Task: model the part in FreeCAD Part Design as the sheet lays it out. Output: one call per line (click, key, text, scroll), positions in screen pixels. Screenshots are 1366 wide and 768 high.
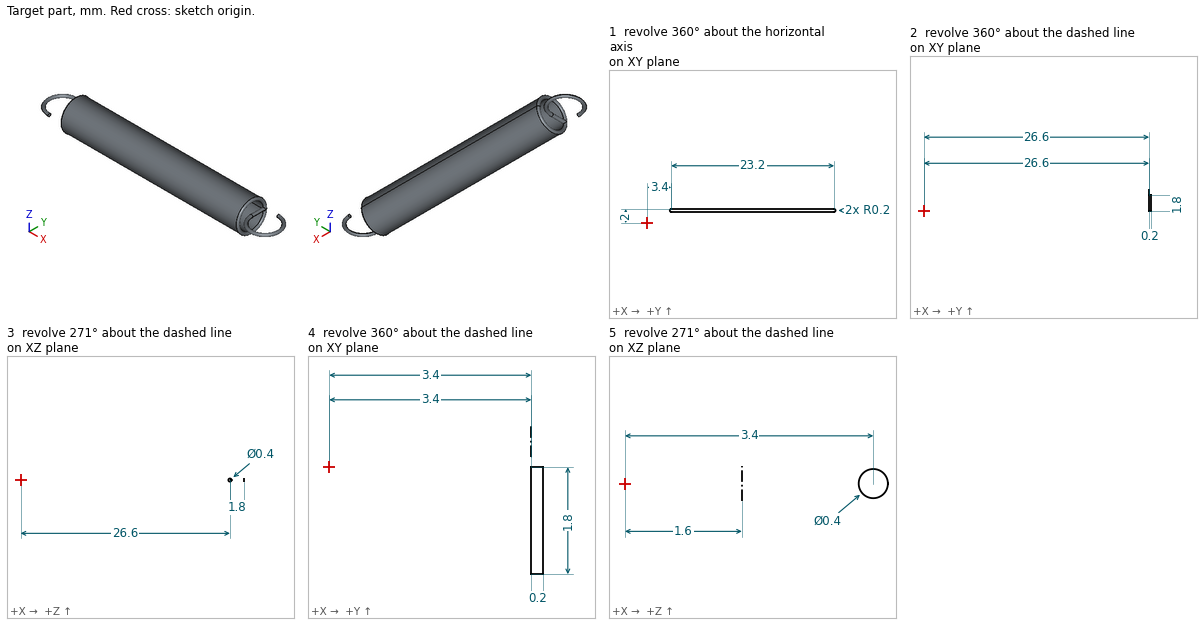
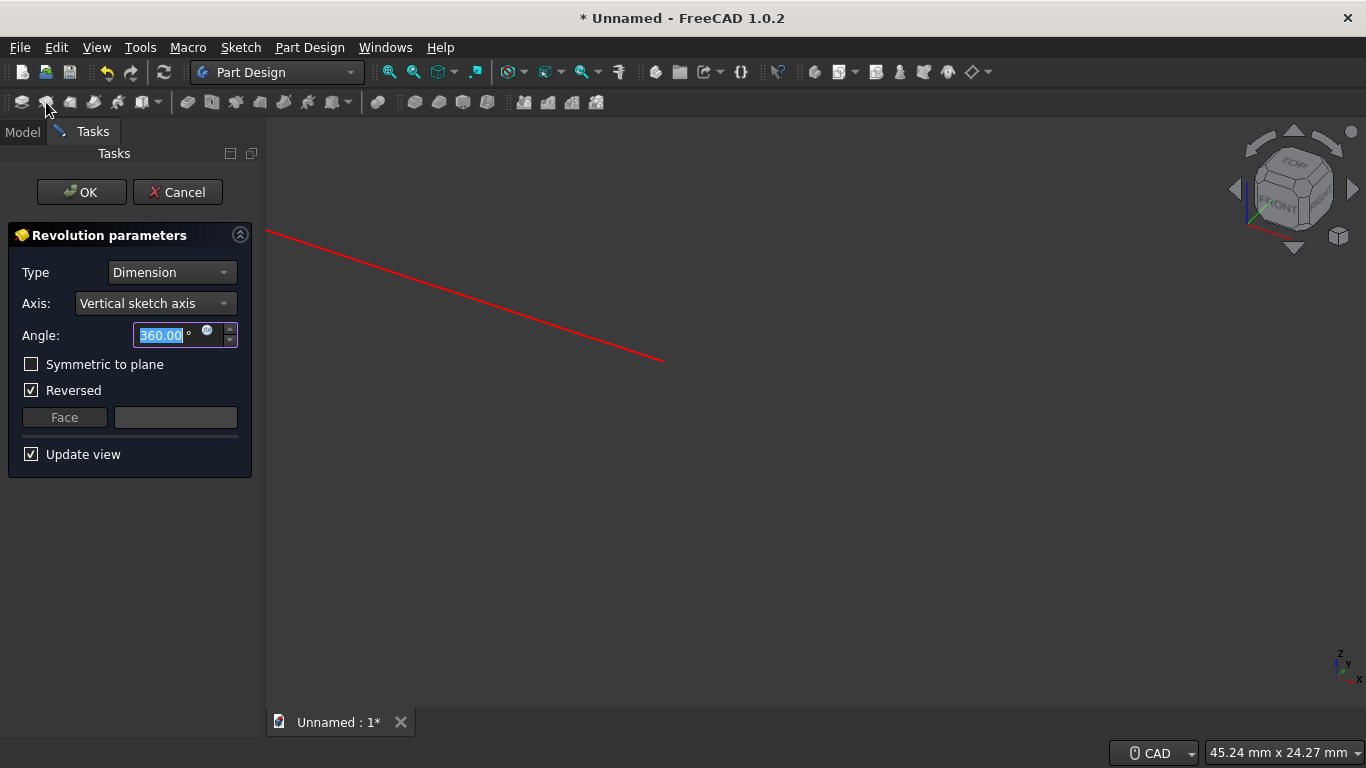
click(156, 304)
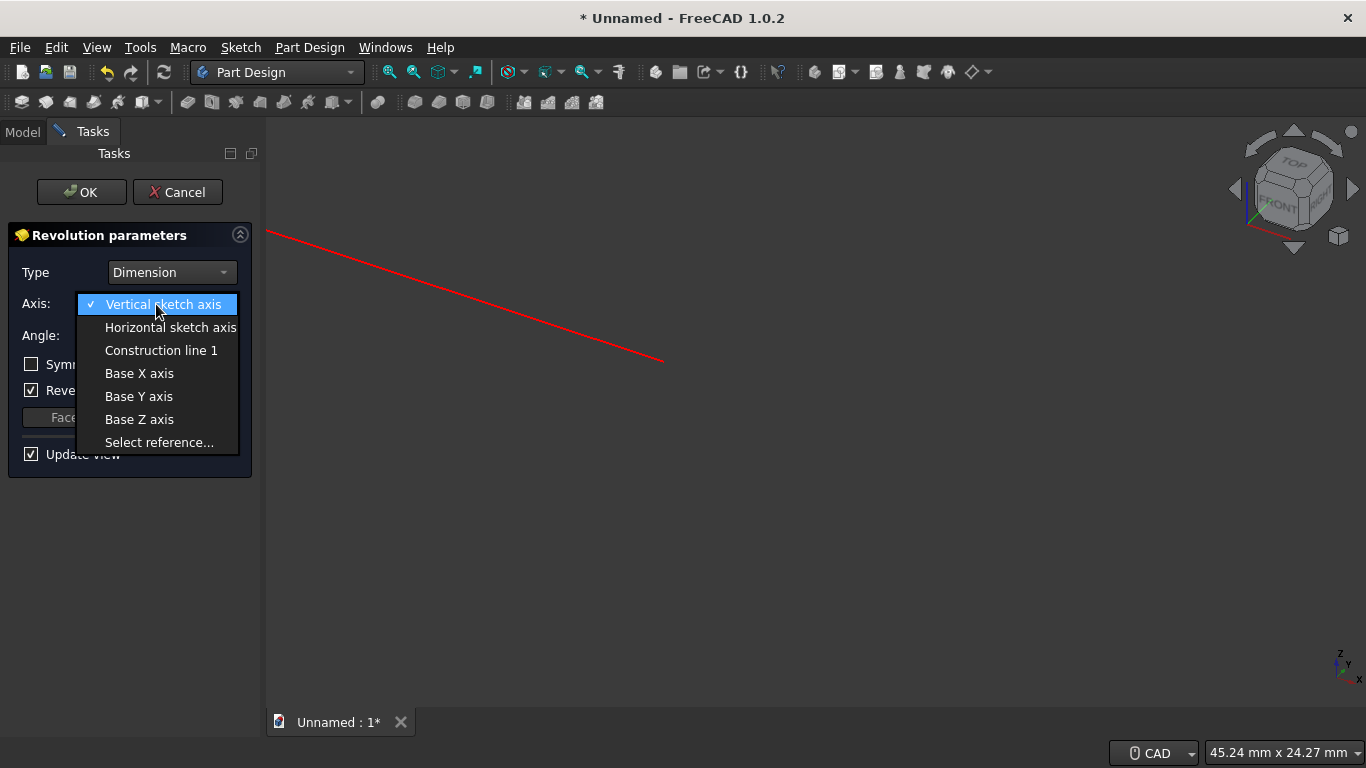
click(156, 350)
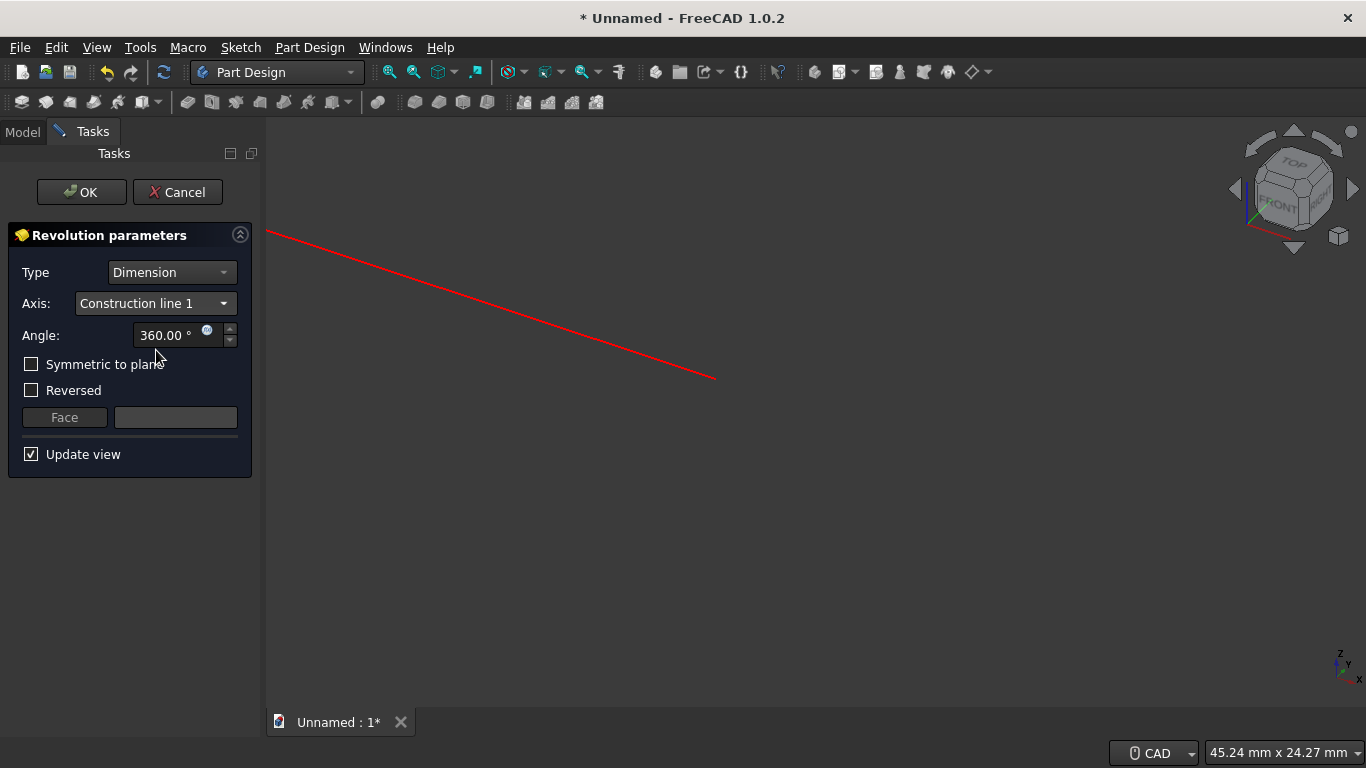
triple_click(178, 335)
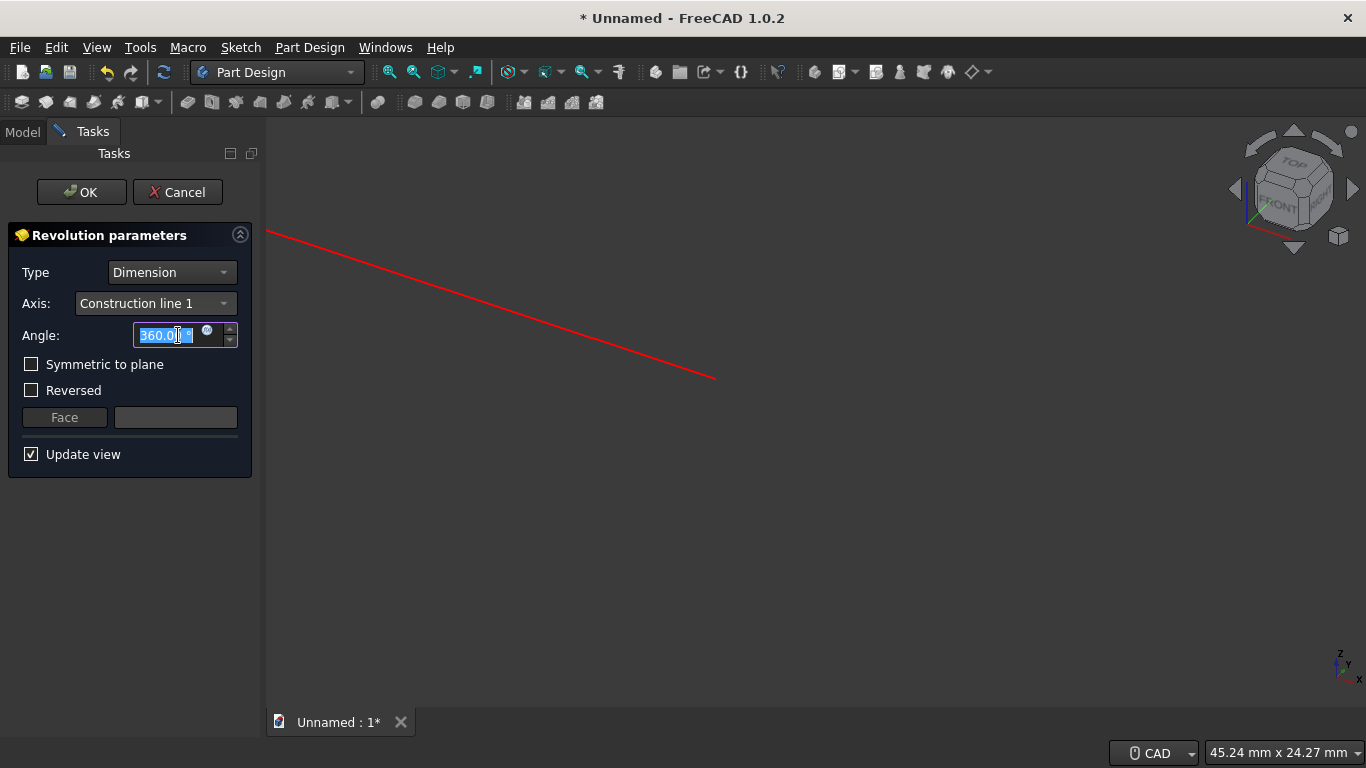
text(271)
key(Tab)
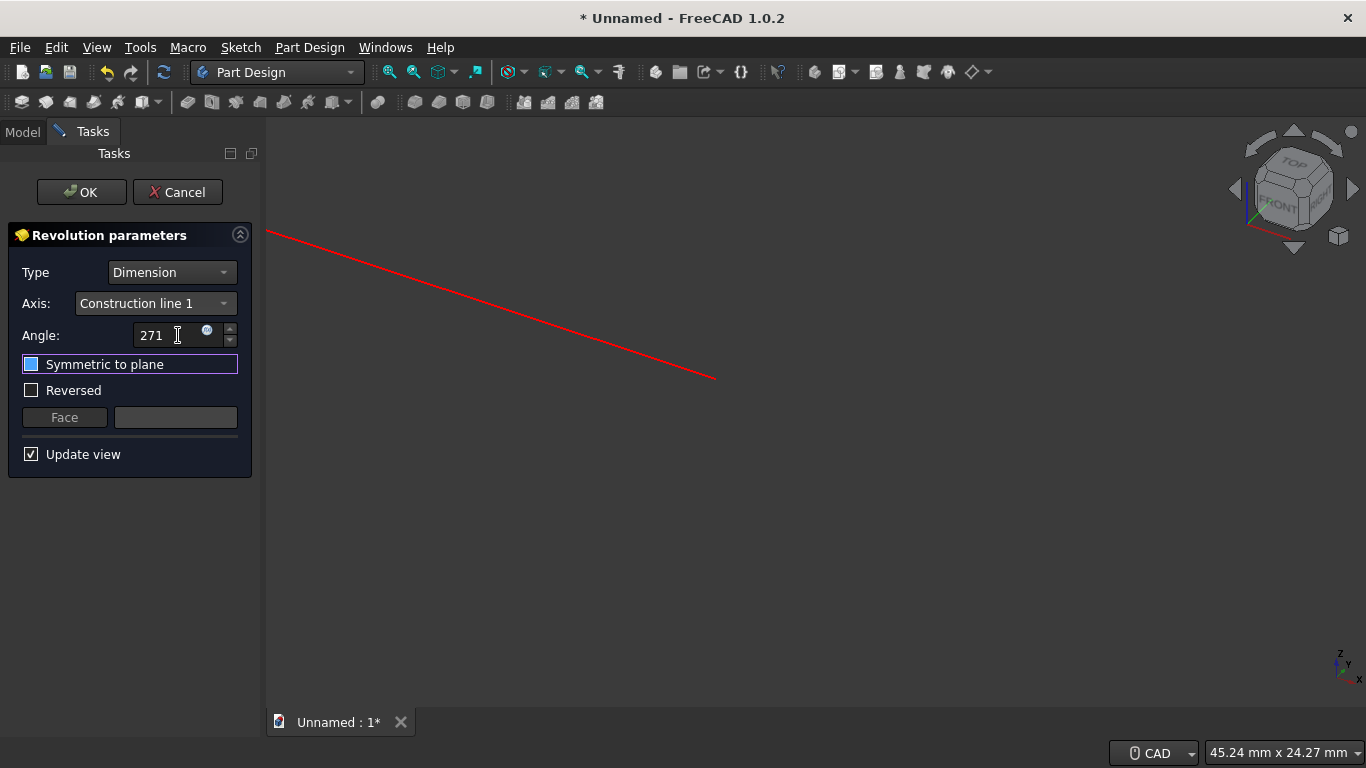
click(82, 192)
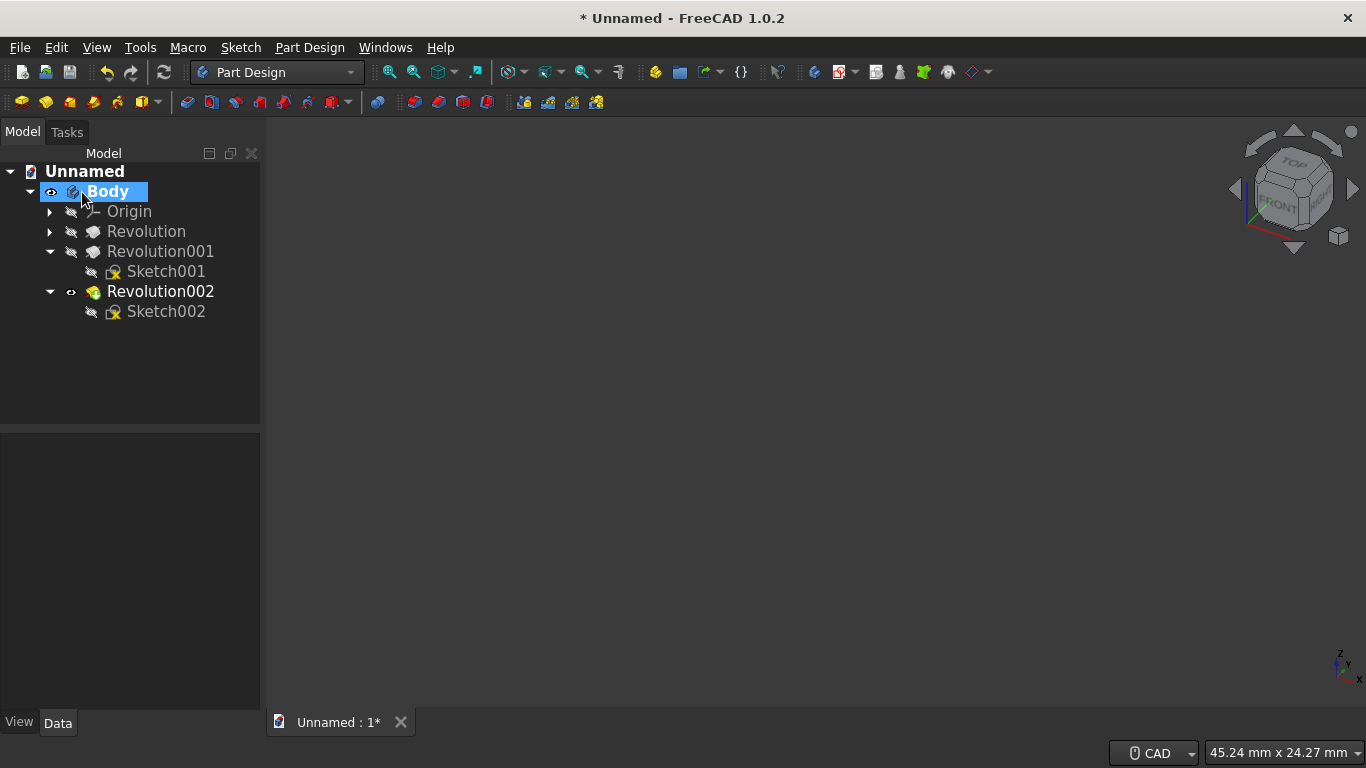
click(390, 72)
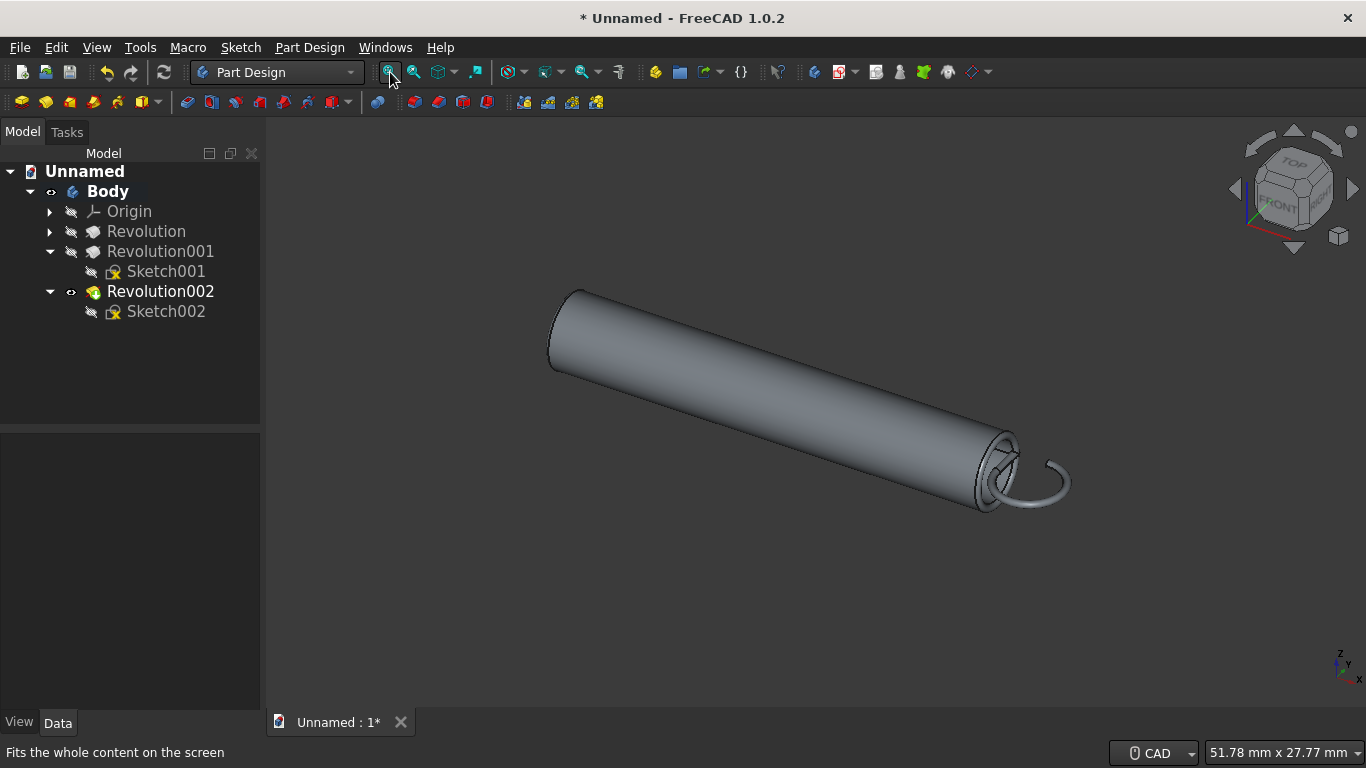
click(840, 72)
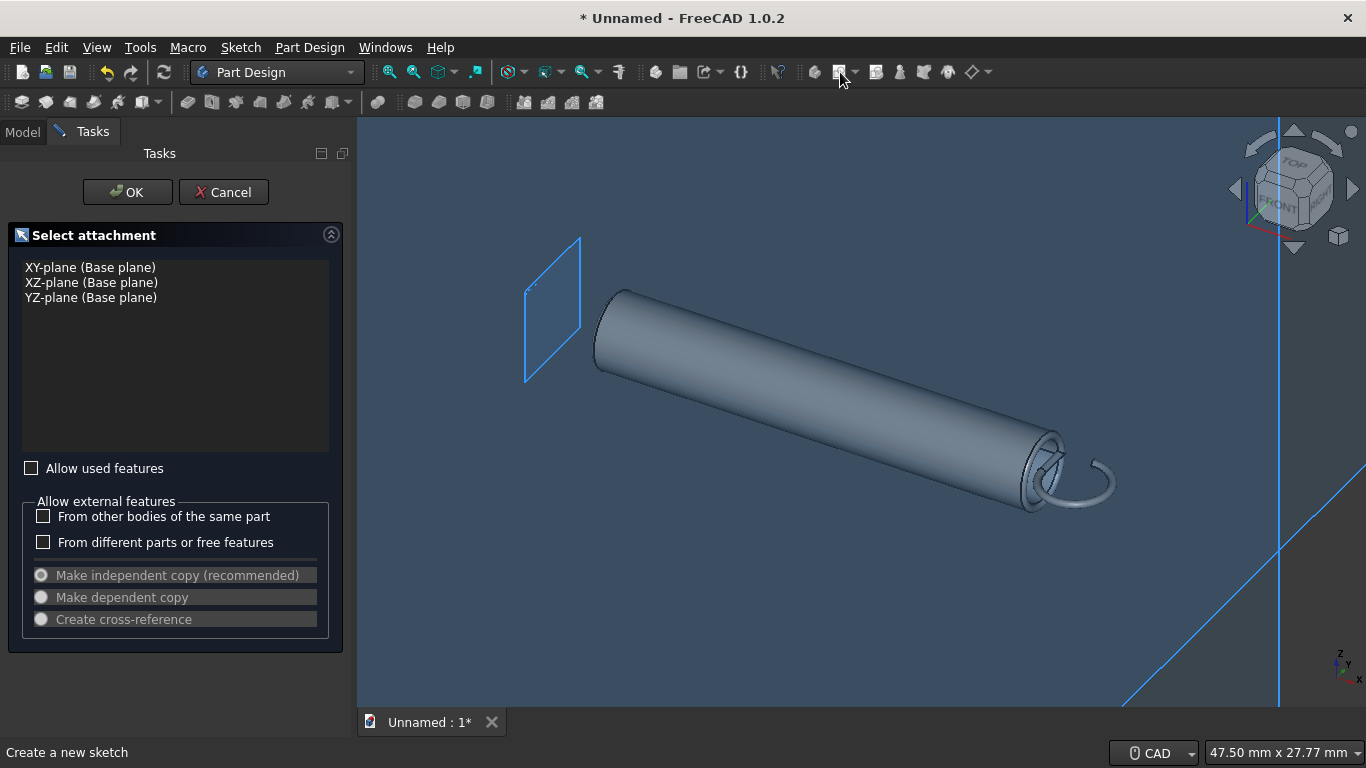
click(82, 268)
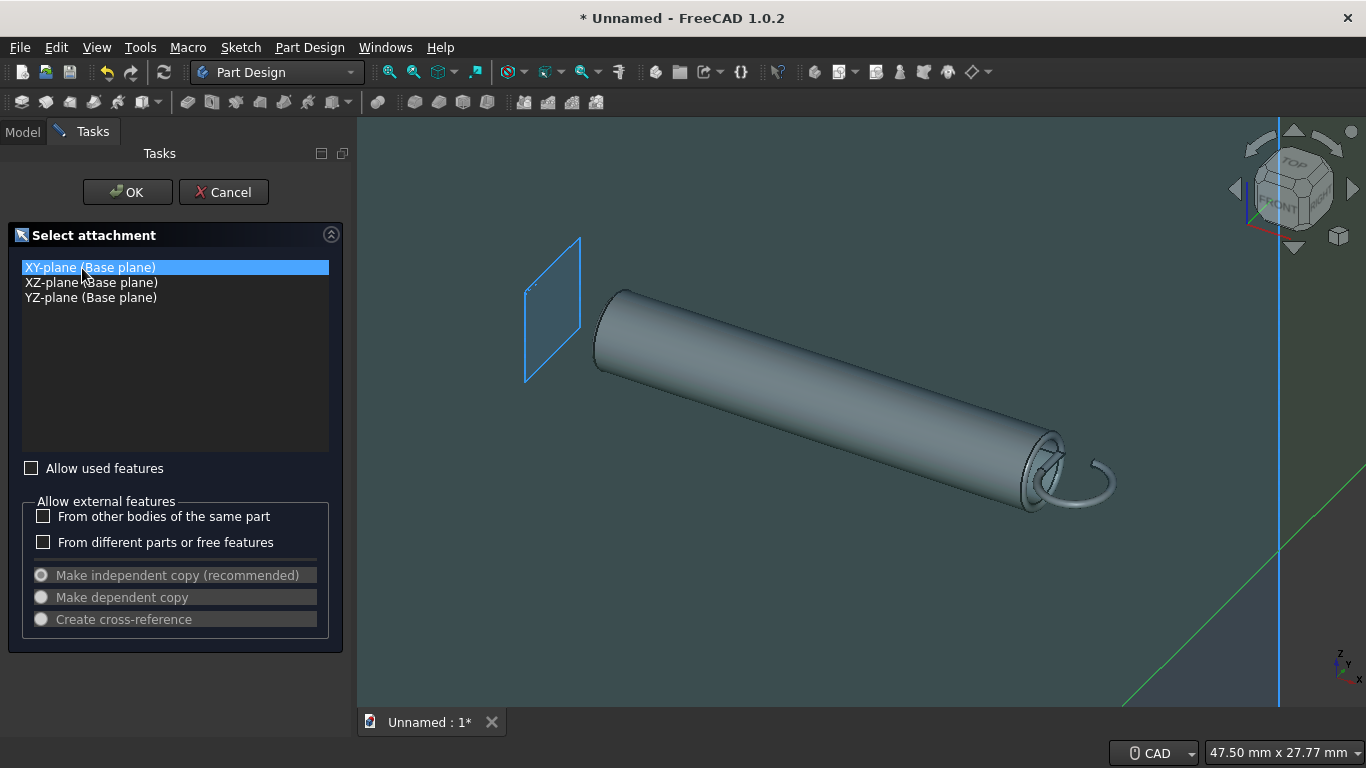
click(128, 192)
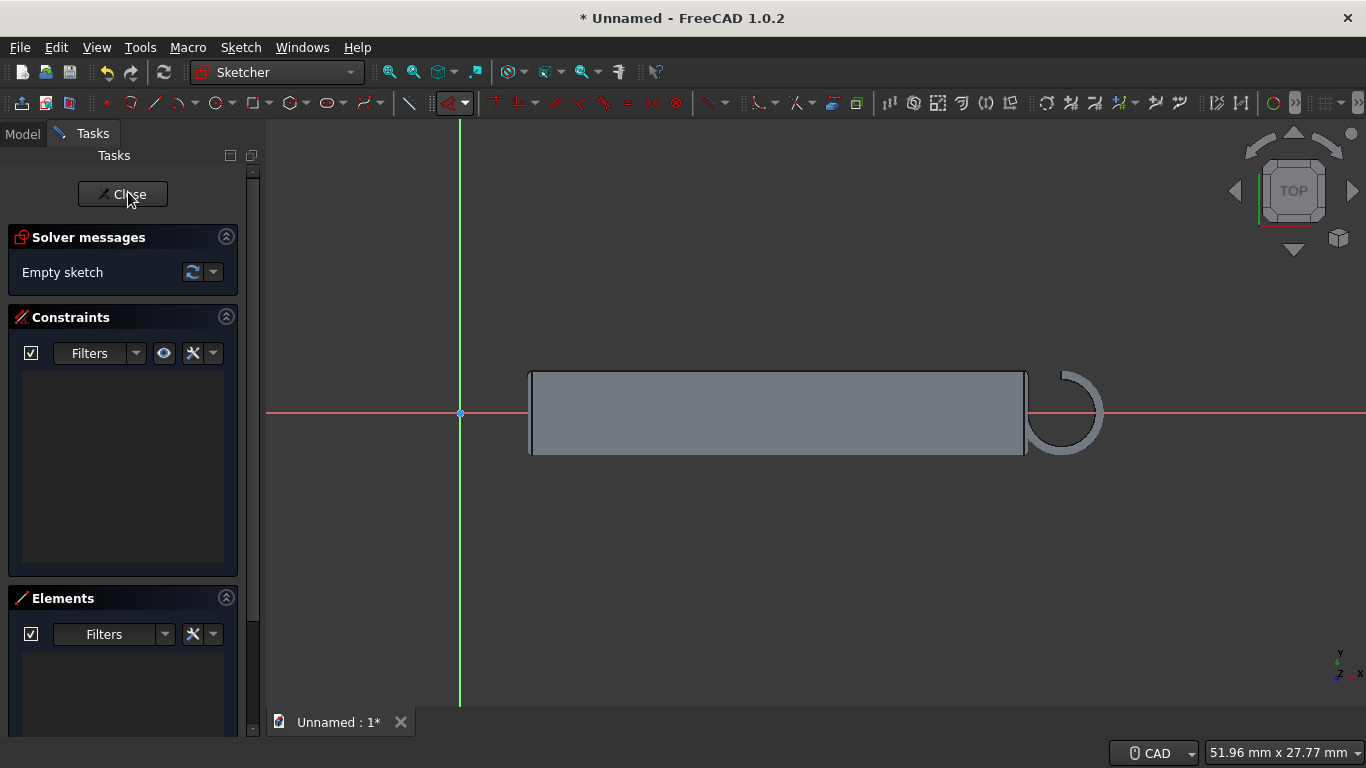
click(70, 104)